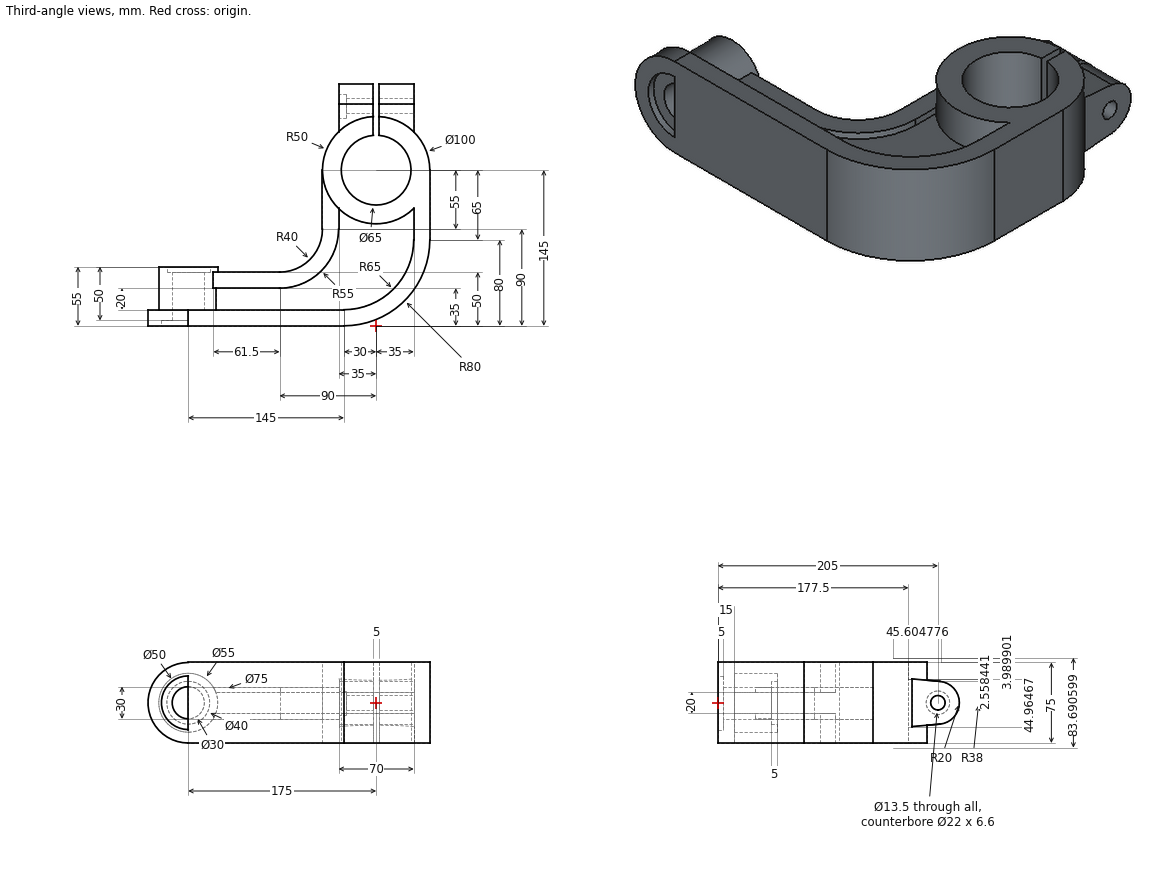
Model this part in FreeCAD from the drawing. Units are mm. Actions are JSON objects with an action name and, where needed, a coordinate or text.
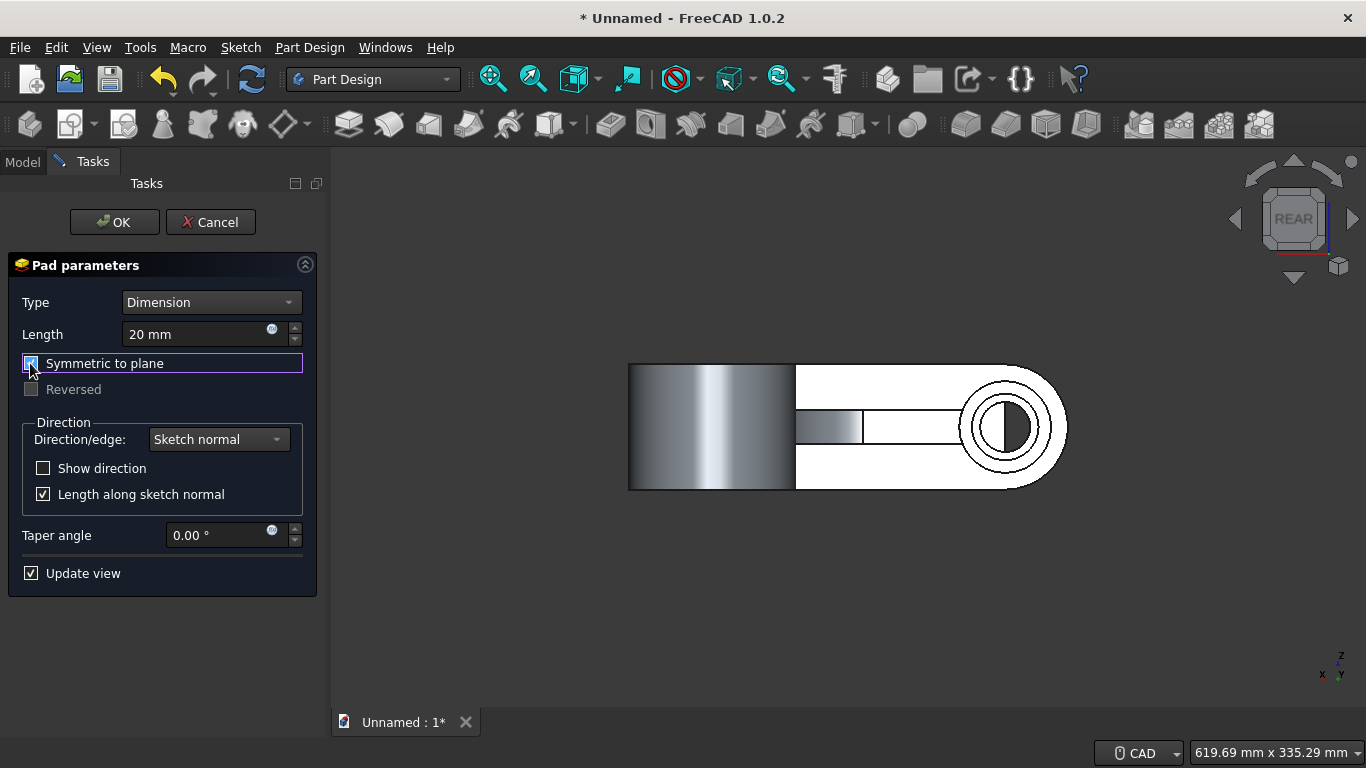
{"action": "left_click", "coordinate": [115, 222]}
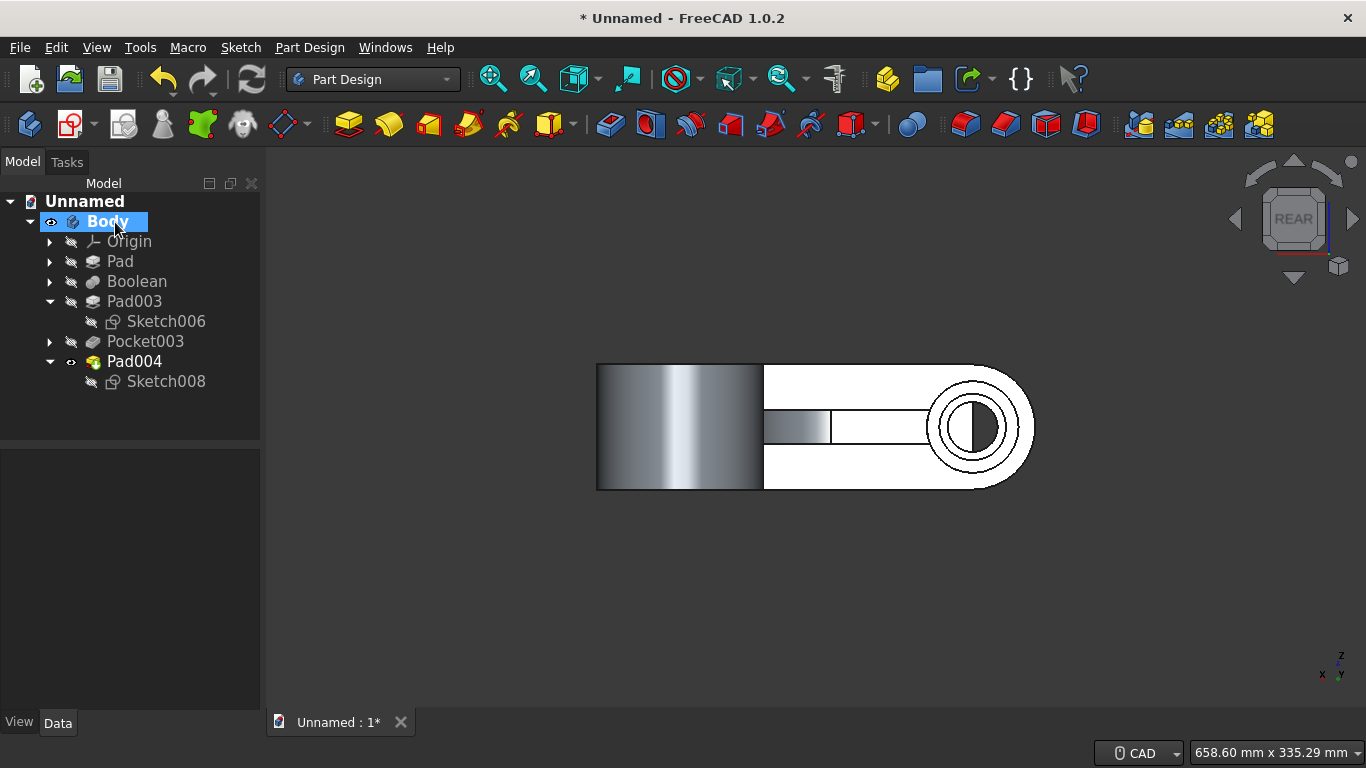
{"action": "key", "text": "v f"}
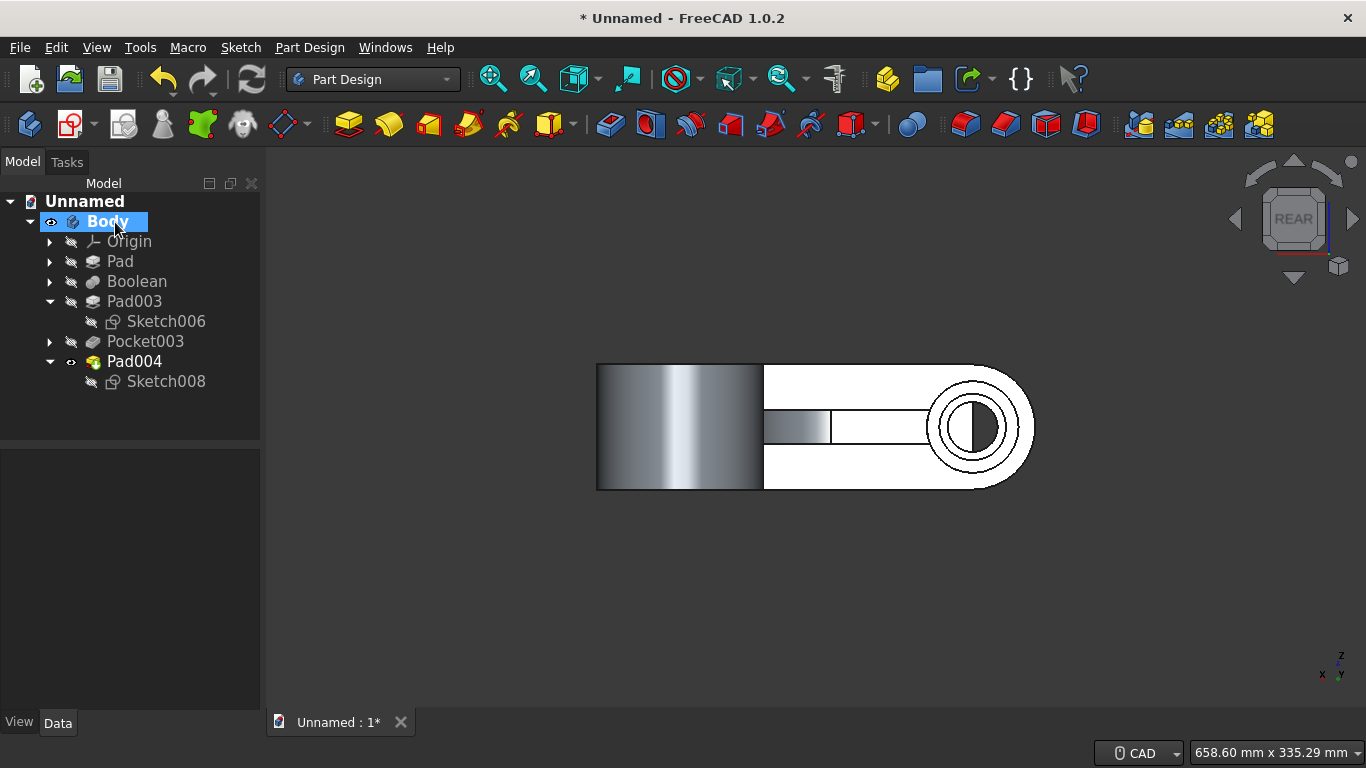
{"action": "left_click", "coordinate": [70, 124]}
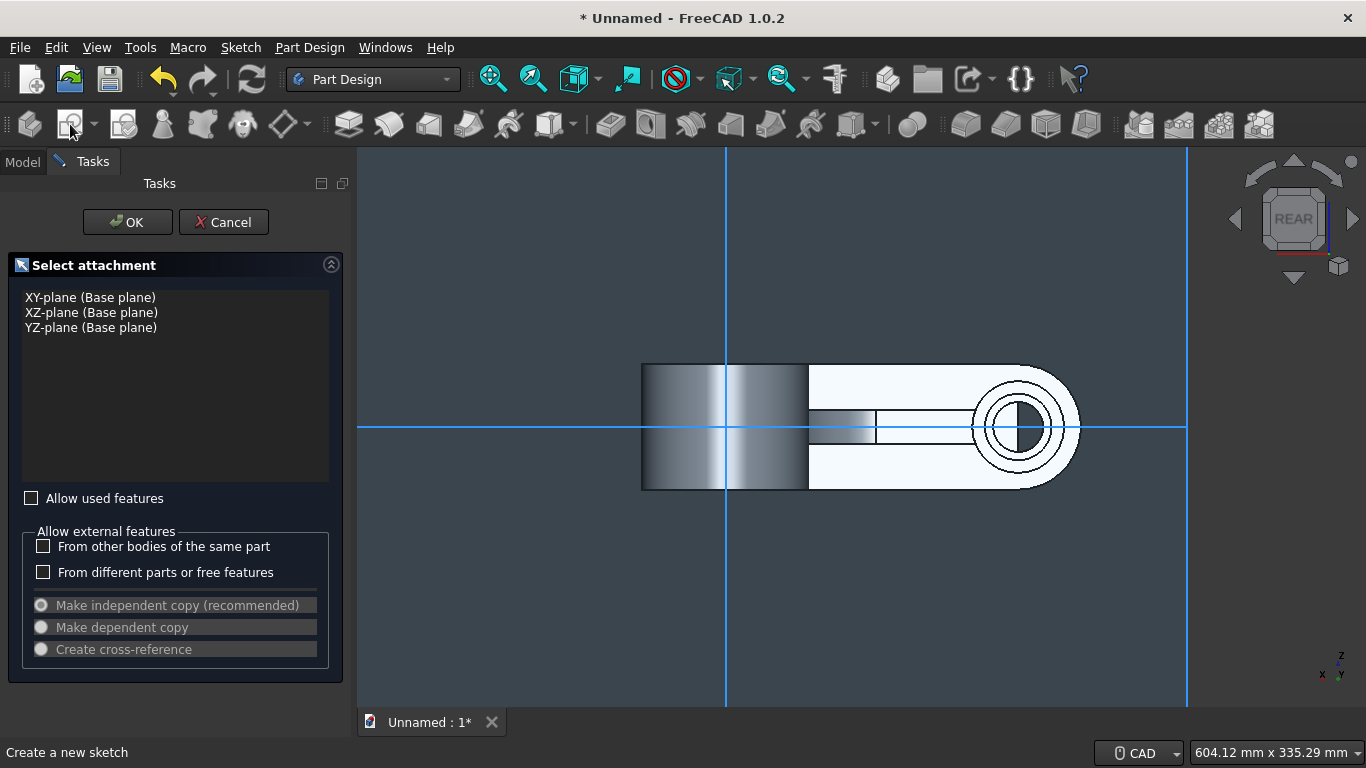
{"action": "left_click", "coordinate": [82, 298]}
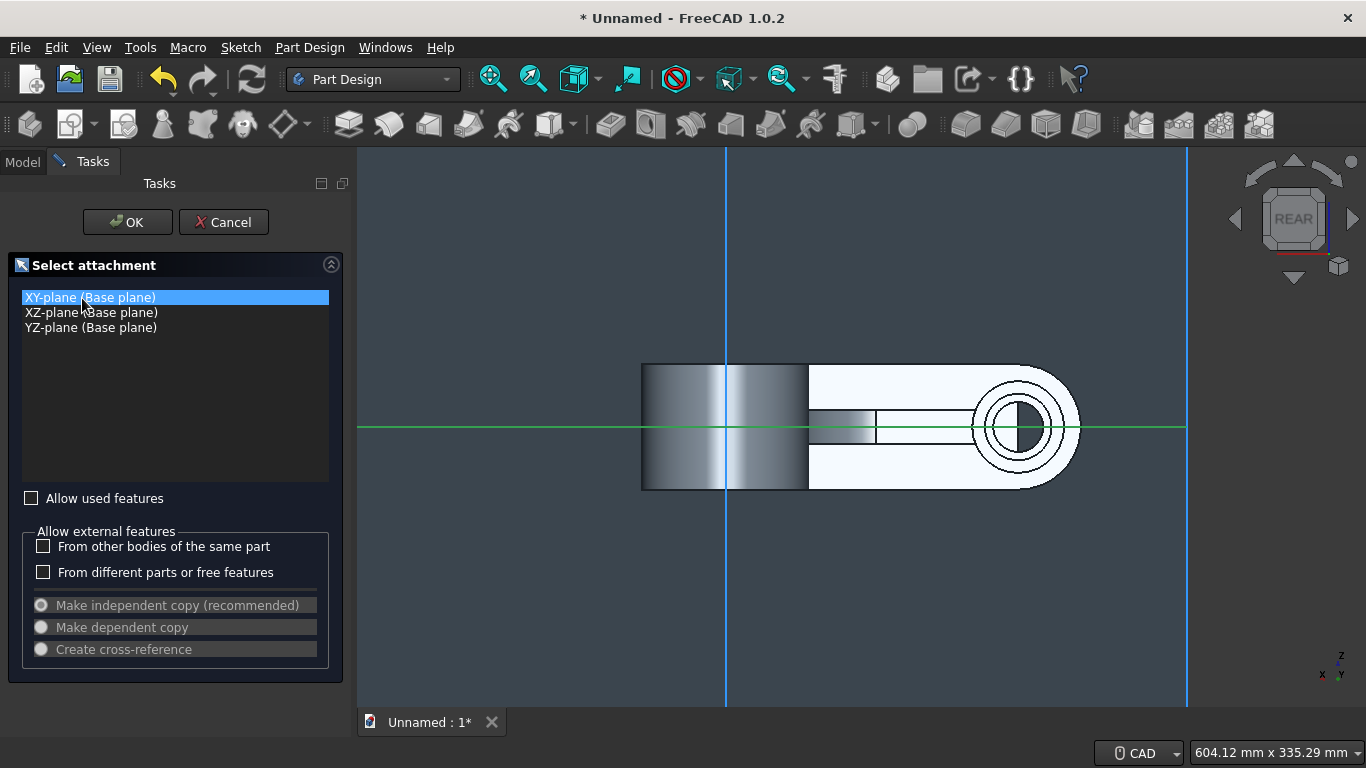
{"action": "left_click", "coordinate": [128, 222]}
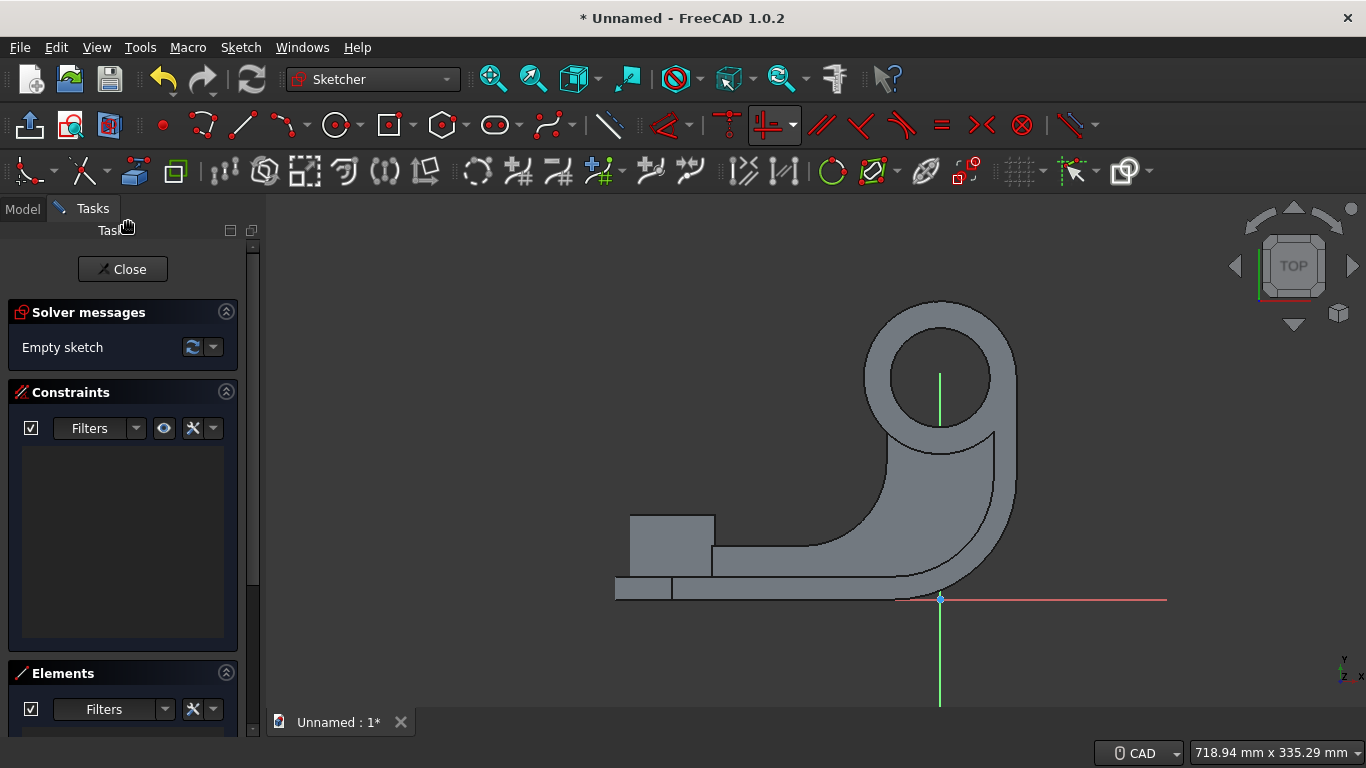
{"action": "left_click", "coordinate": [110, 126]}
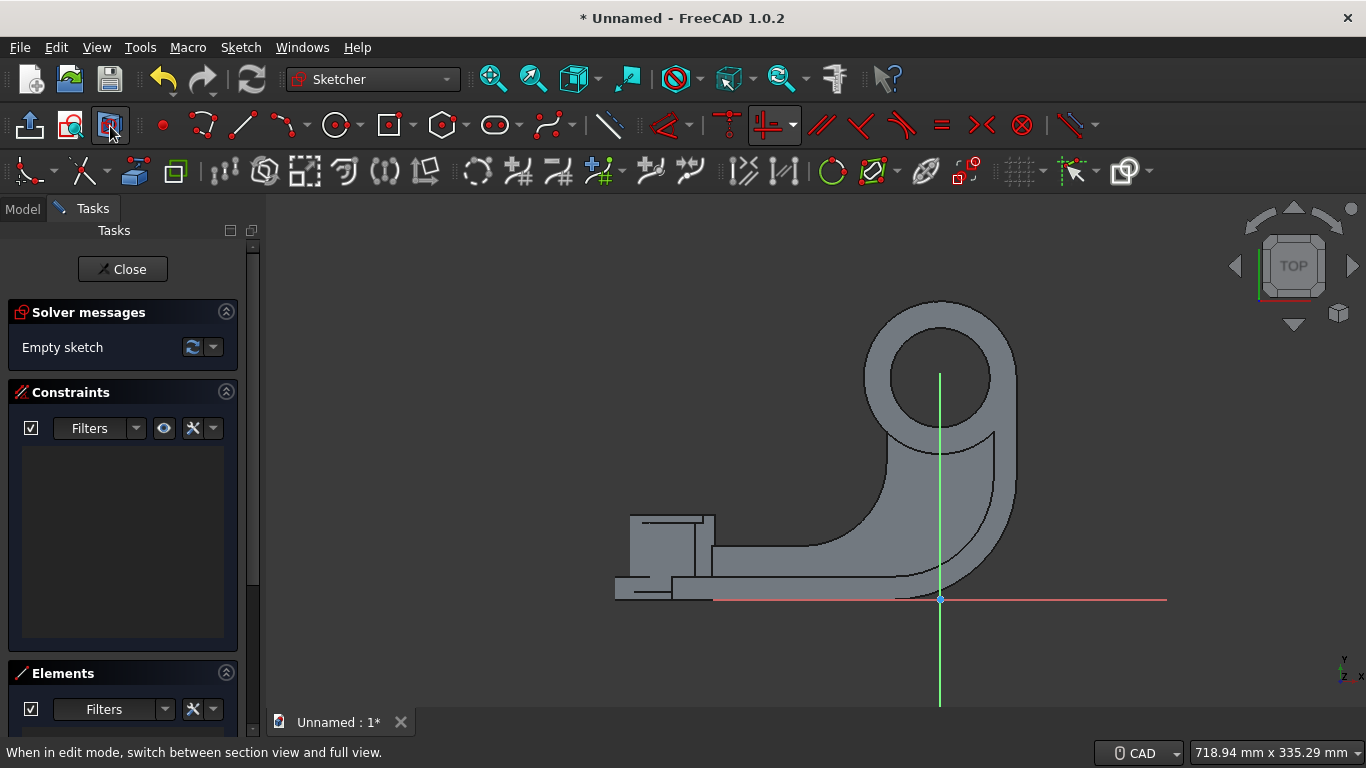
{"action": "scroll", "coordinate": [980, 566], "scroll_direction": "up", "scroll_amount": 2}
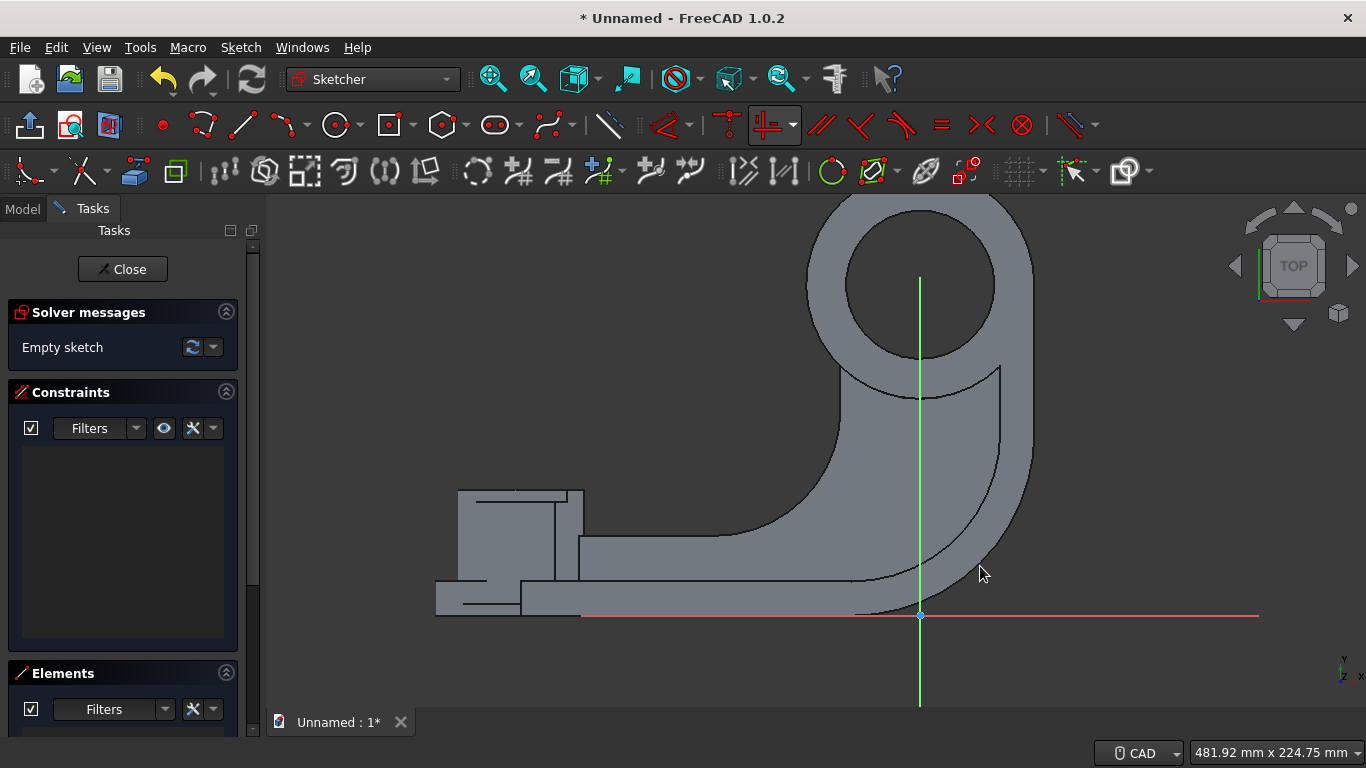
{"action": "left_click", "coordinate": [244, 126]}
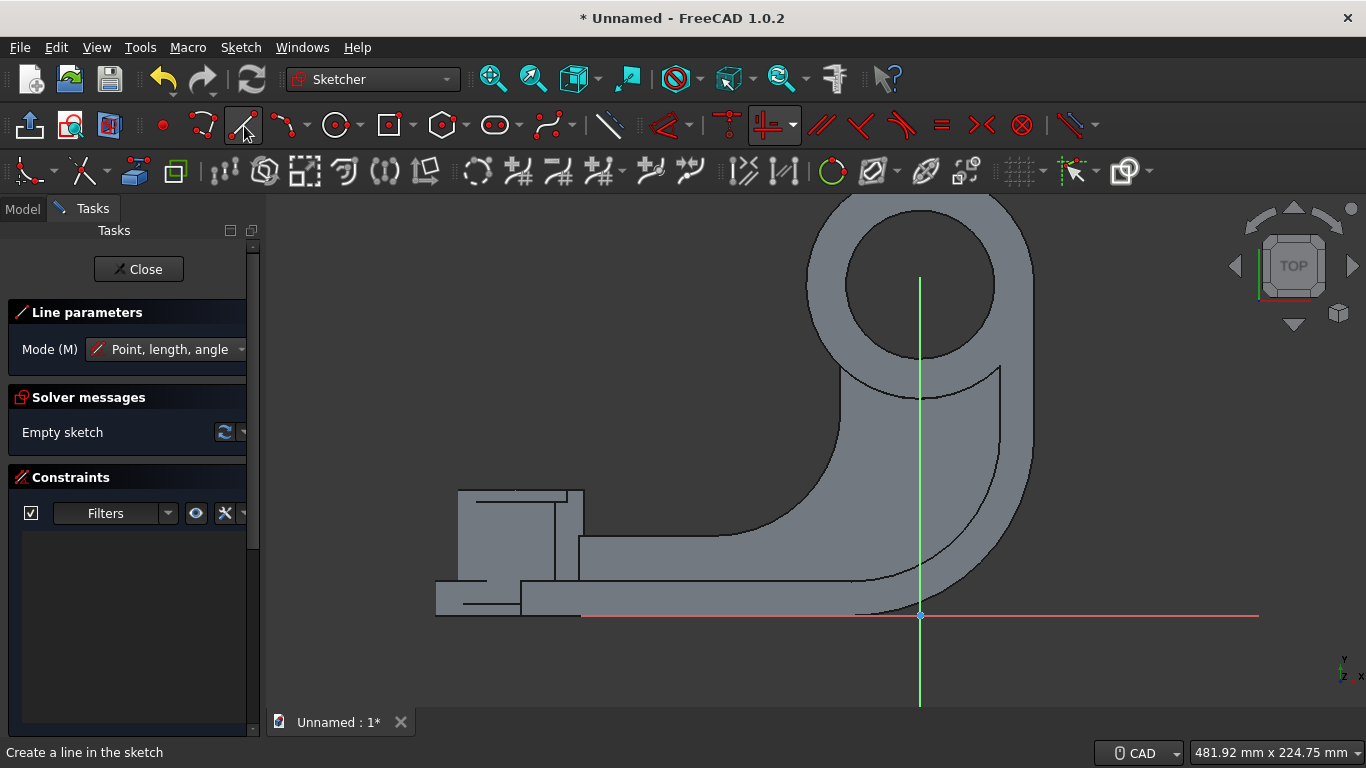
{"action": "left_click", "coordinate": [840, 410]}
{"action": "left_click", "coordinate": [840, 366]}